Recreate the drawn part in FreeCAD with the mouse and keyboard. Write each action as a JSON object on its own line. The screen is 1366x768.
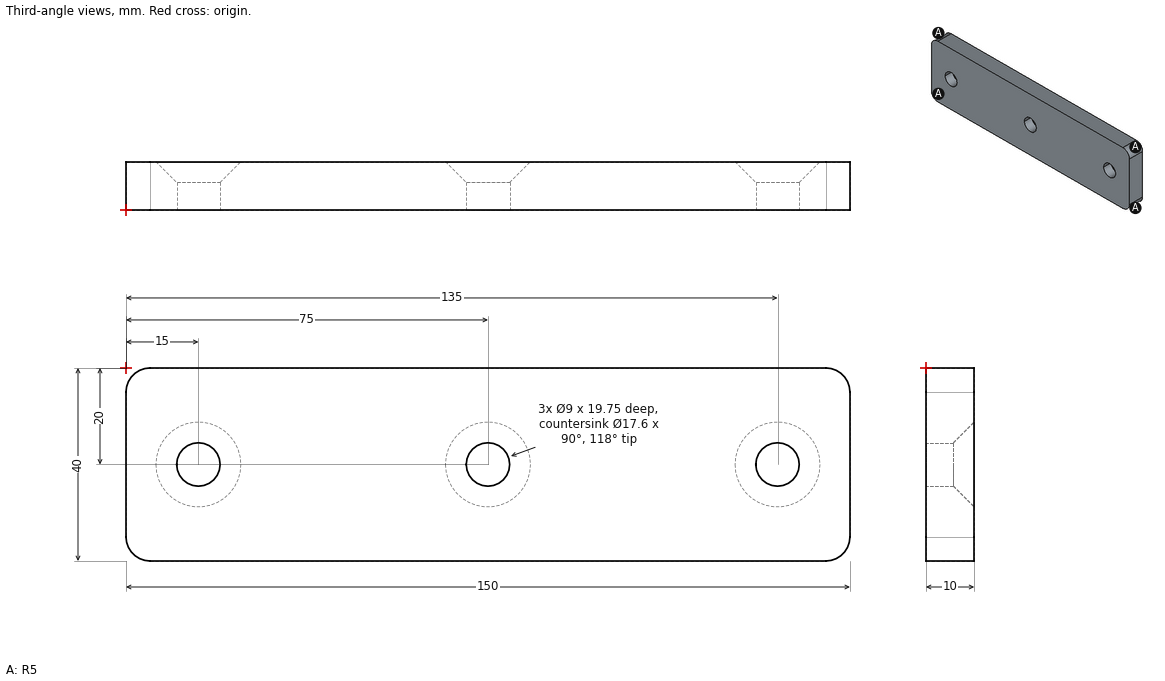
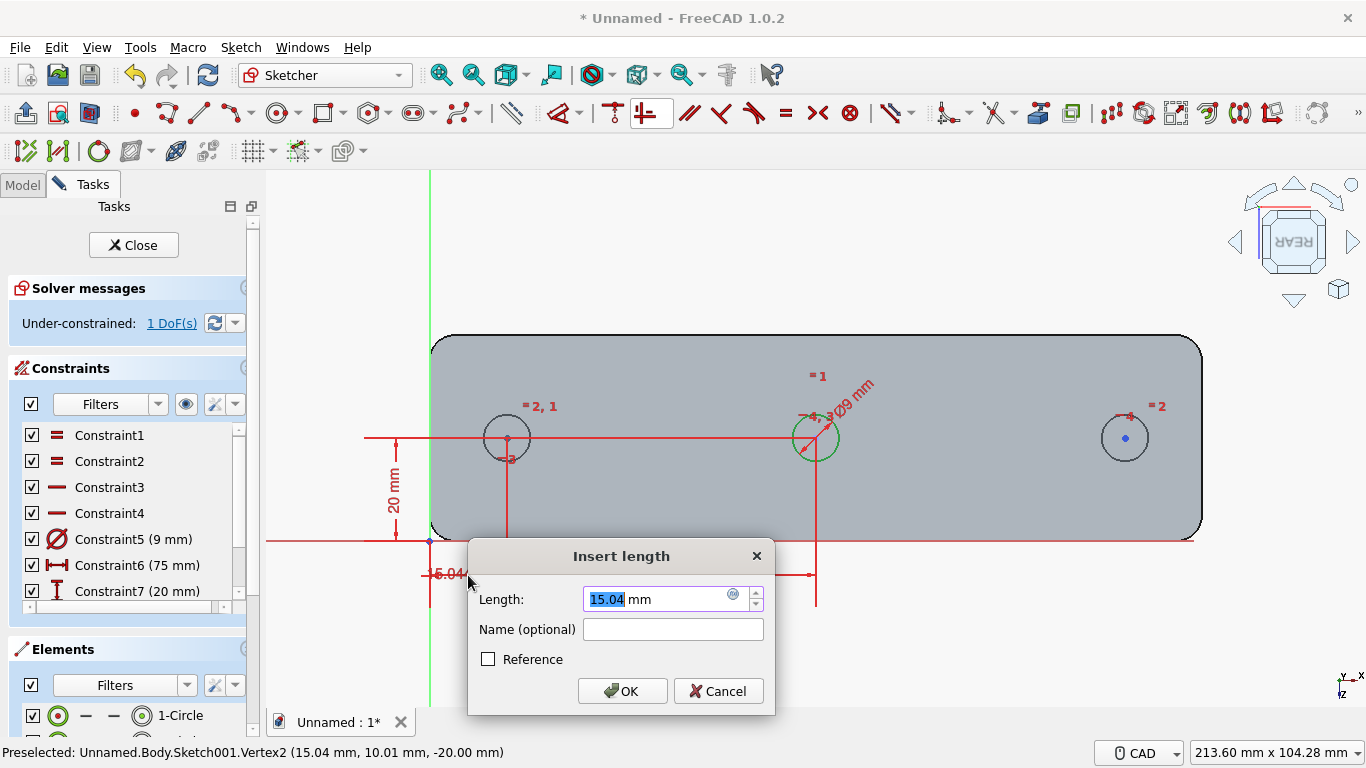
{"action": "type", "text": "15"}
{"action": "key", "text": "Return"}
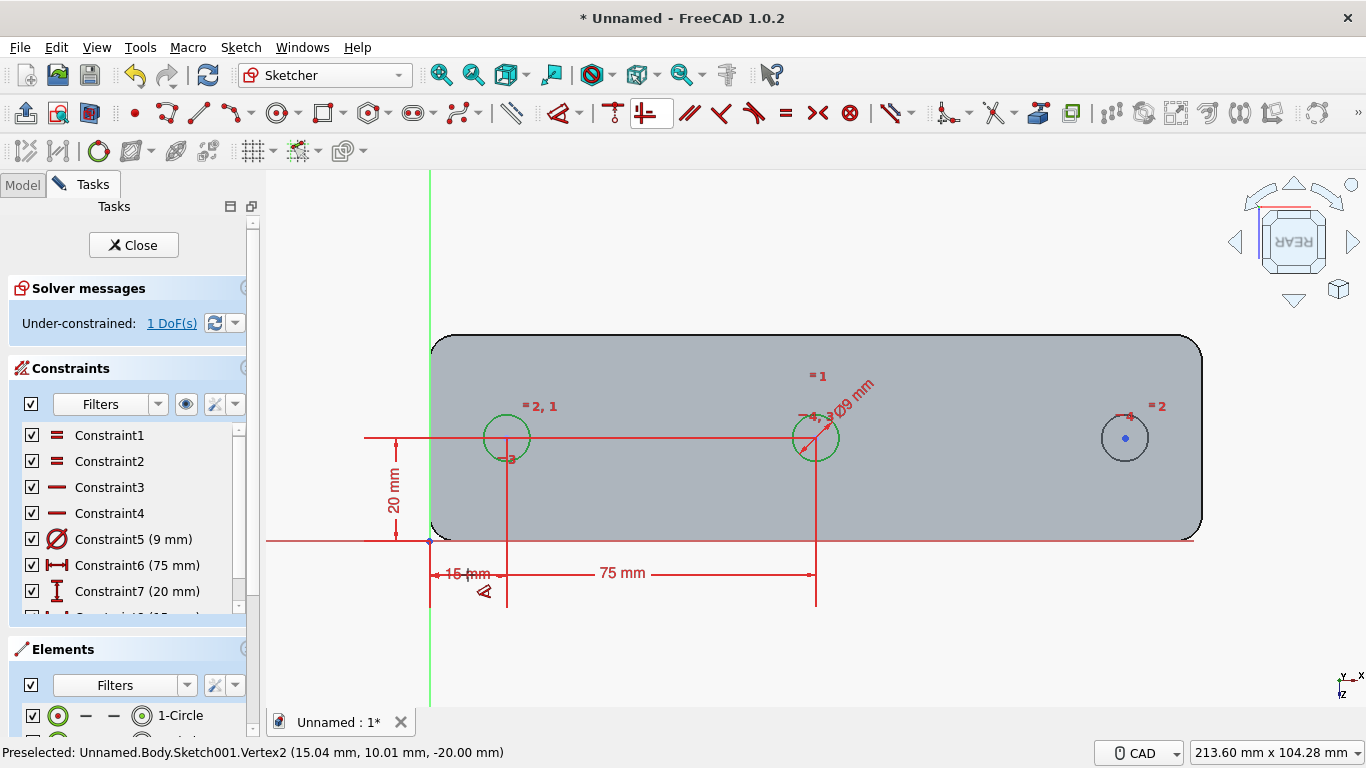
{"action": "left_click", "coordinate": [1125, 438]}
{"action": "left_click", "coordinate": [777, 575]}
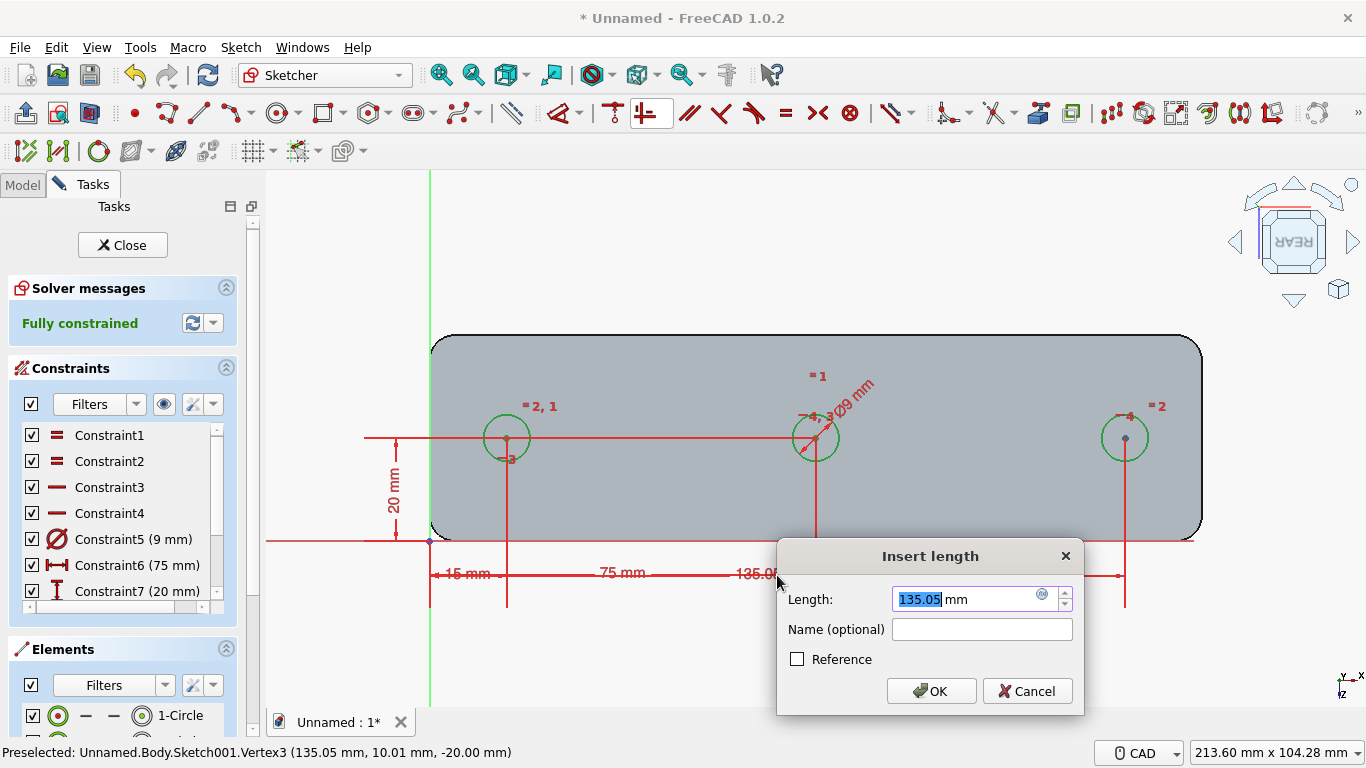
{"action": "type", "text": "135"}
{"action": "key", "text": "Return"}
{"action": "key", "text": "Escape"}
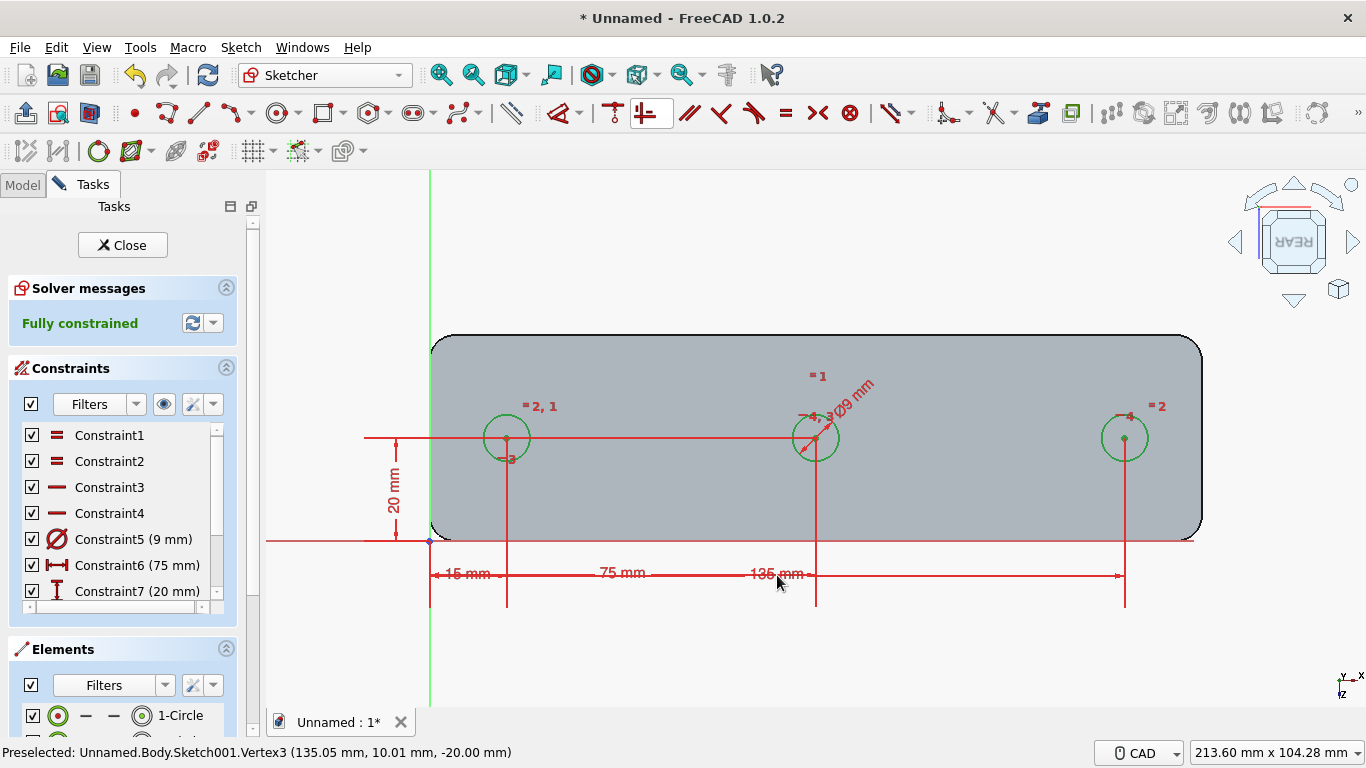
{"action": "left_click", "coordinate": [123, 245]}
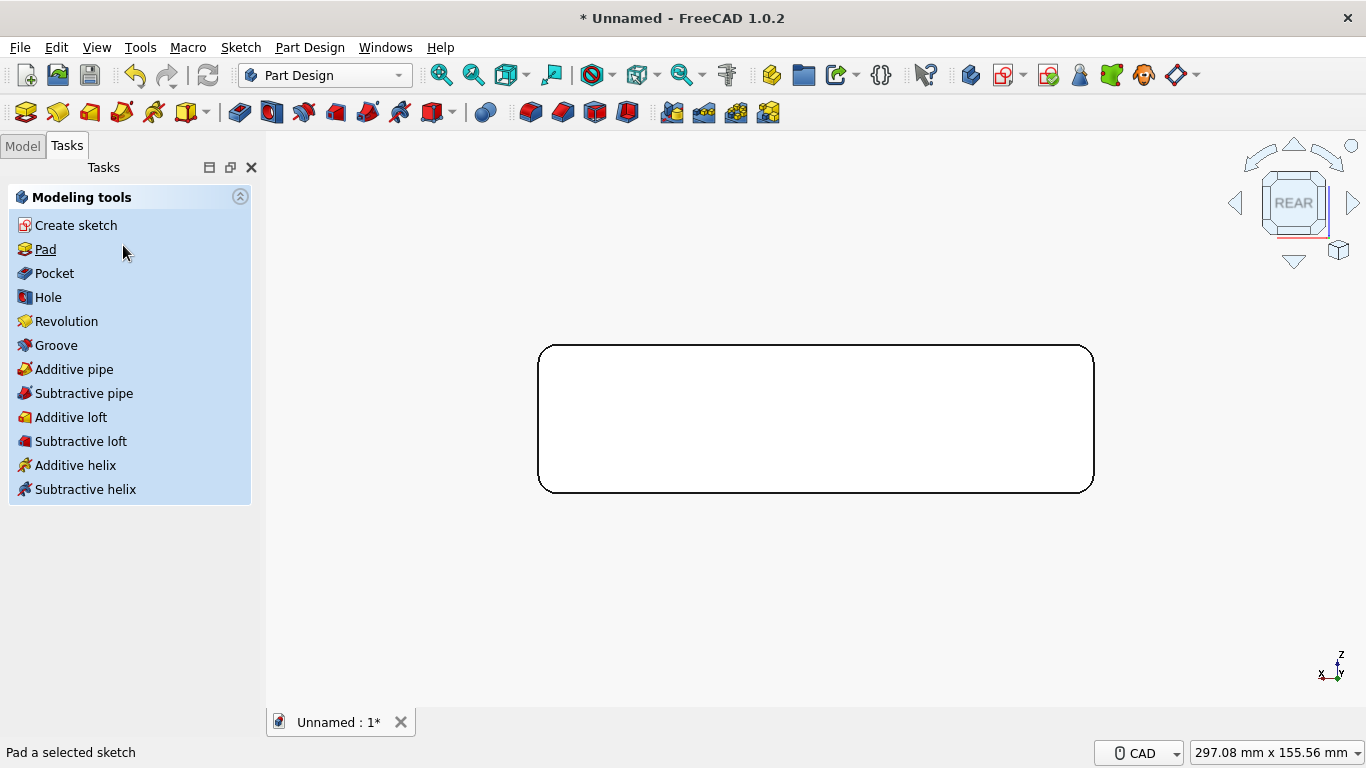
{"action": "left_click", "coordinate": [272, 112]}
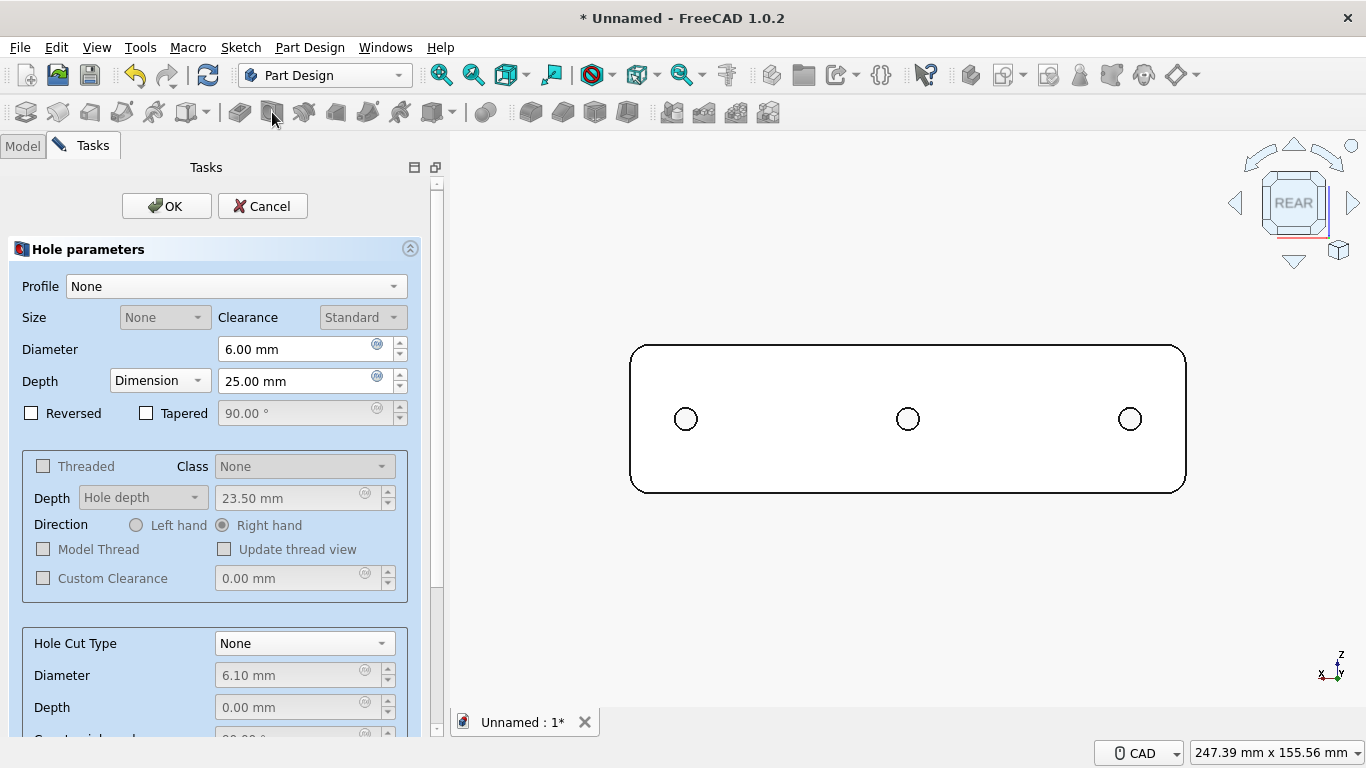
{"action": "triple_click", "coordinate": [305, 349]}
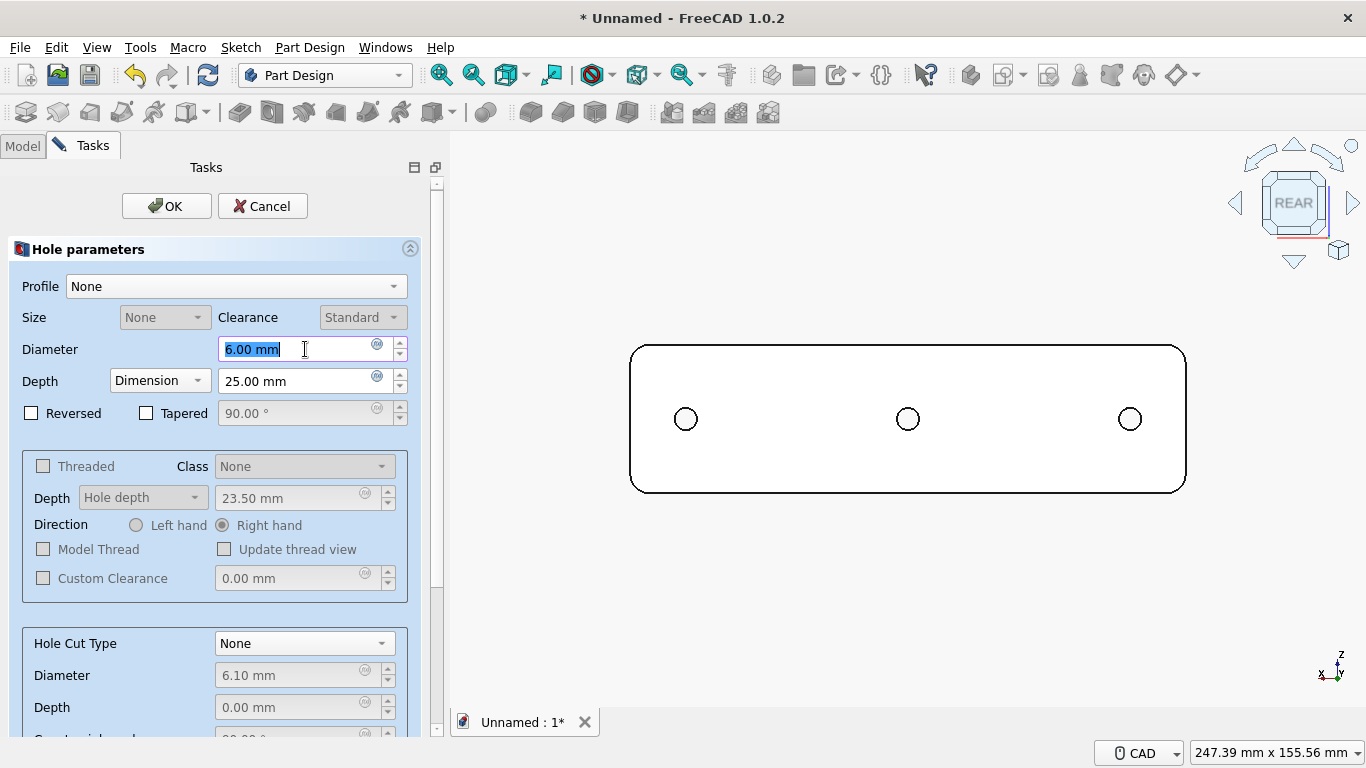
{"action": "type", "text": "9"}
{"action": "key", "text": "Tab"}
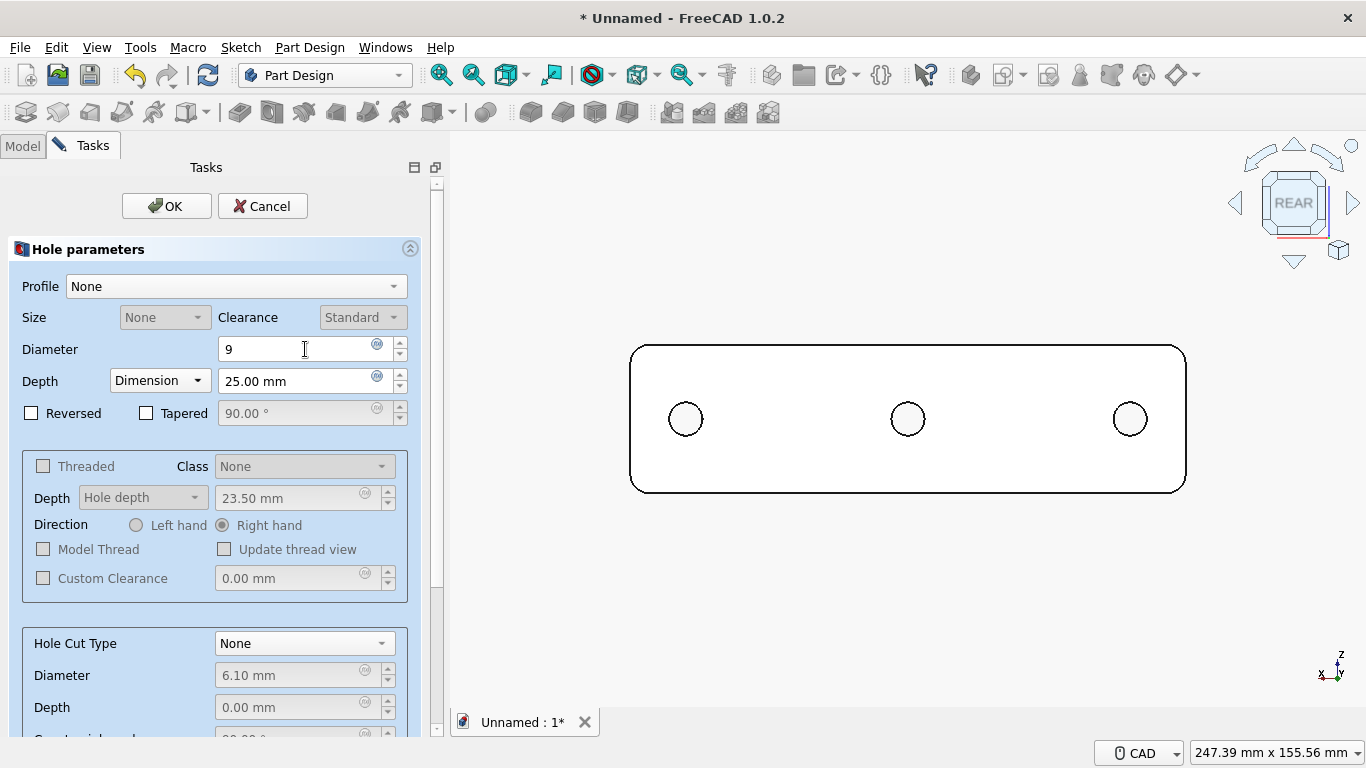
{"action": "triple_click", "coordinate": [305, 381]}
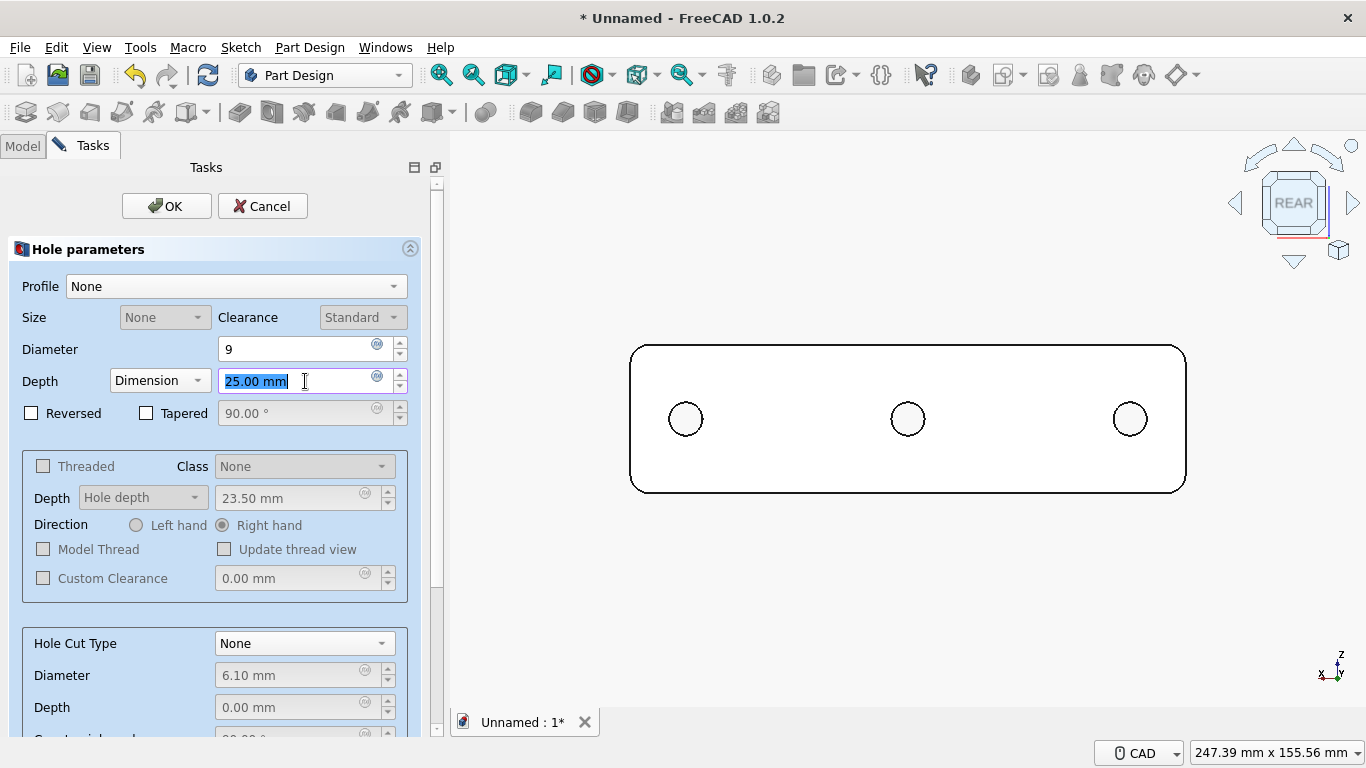
{"action": "type", "text": "19.75"}
{"action": "key", "text": "Tab"}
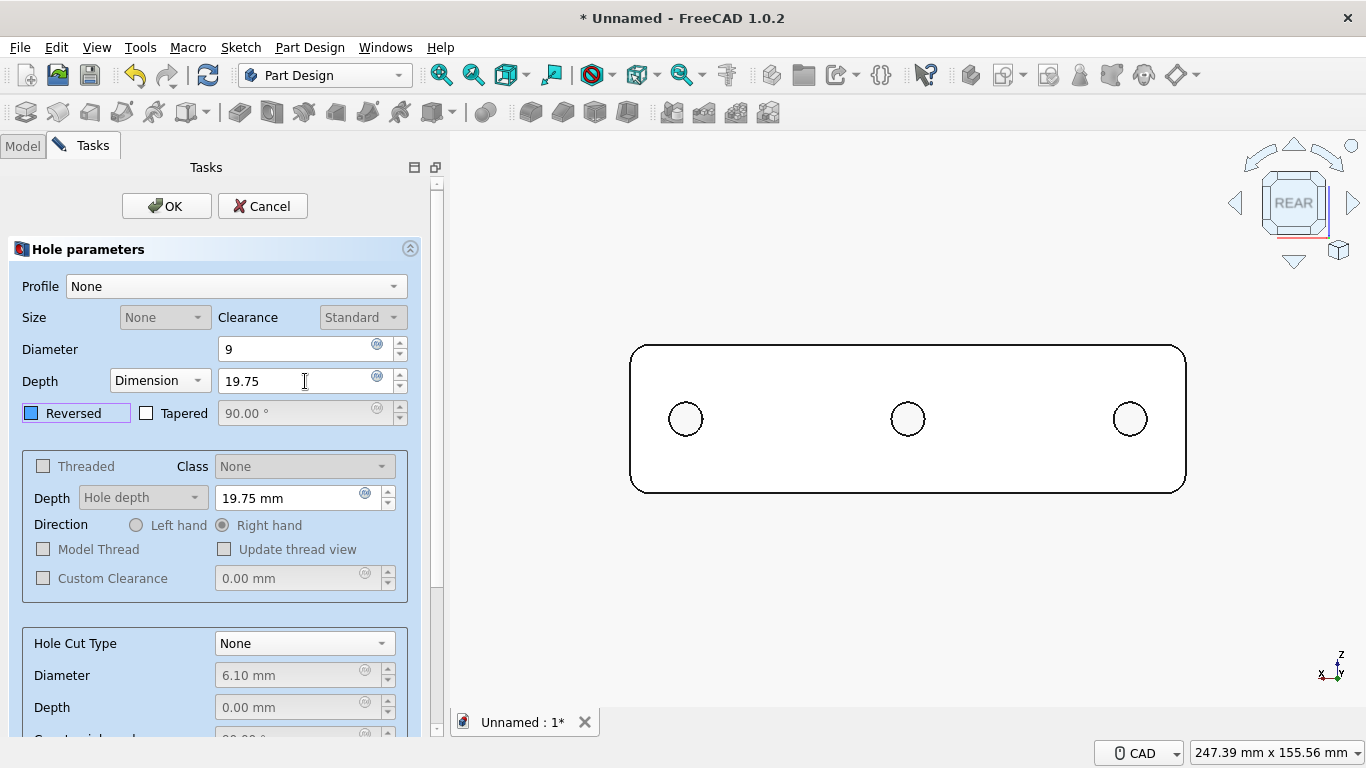
{"action": "left_click", "coordinate": [306, 644]}